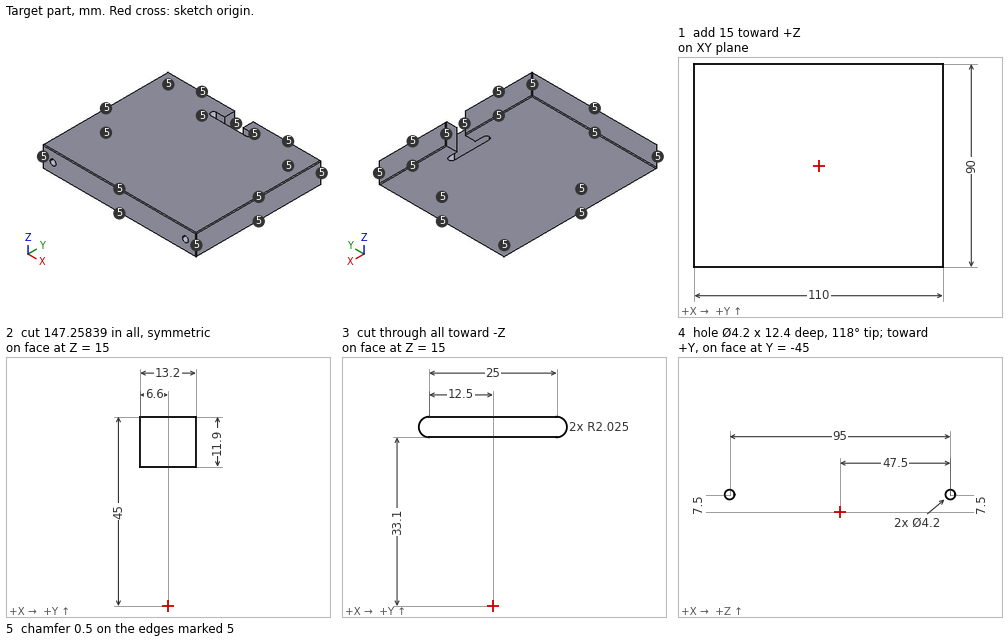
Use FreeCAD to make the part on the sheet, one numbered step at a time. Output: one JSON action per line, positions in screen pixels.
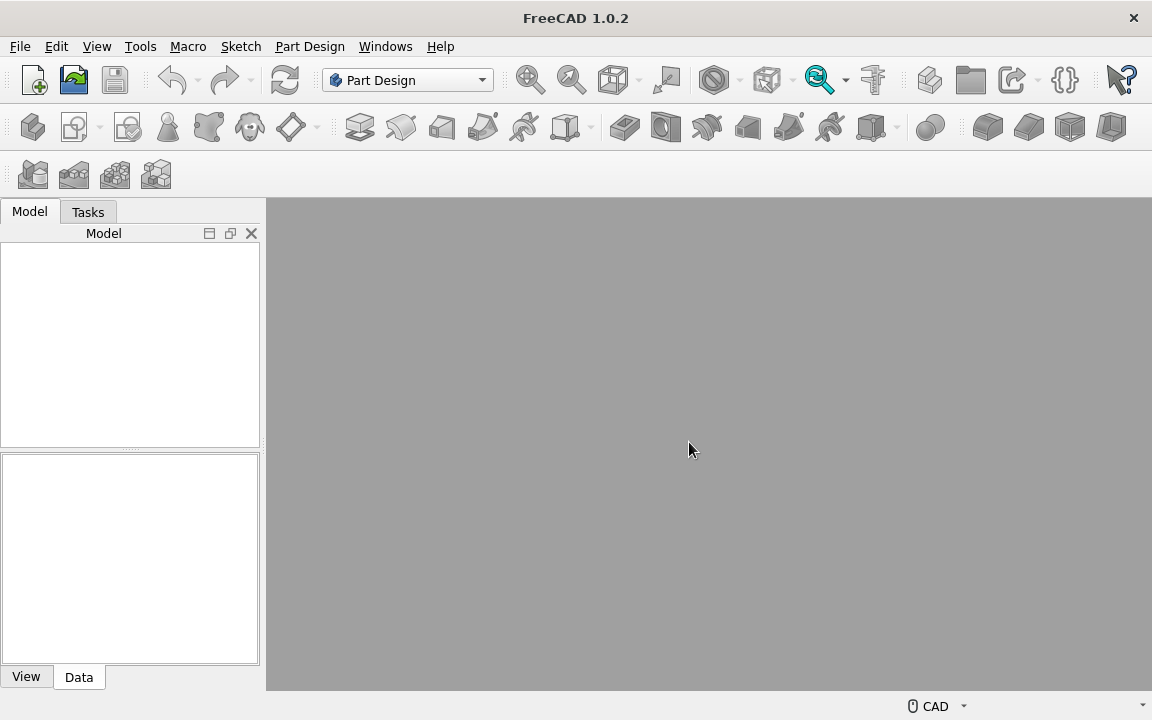
{"action": "left_click", "coordinate": [33, 80]}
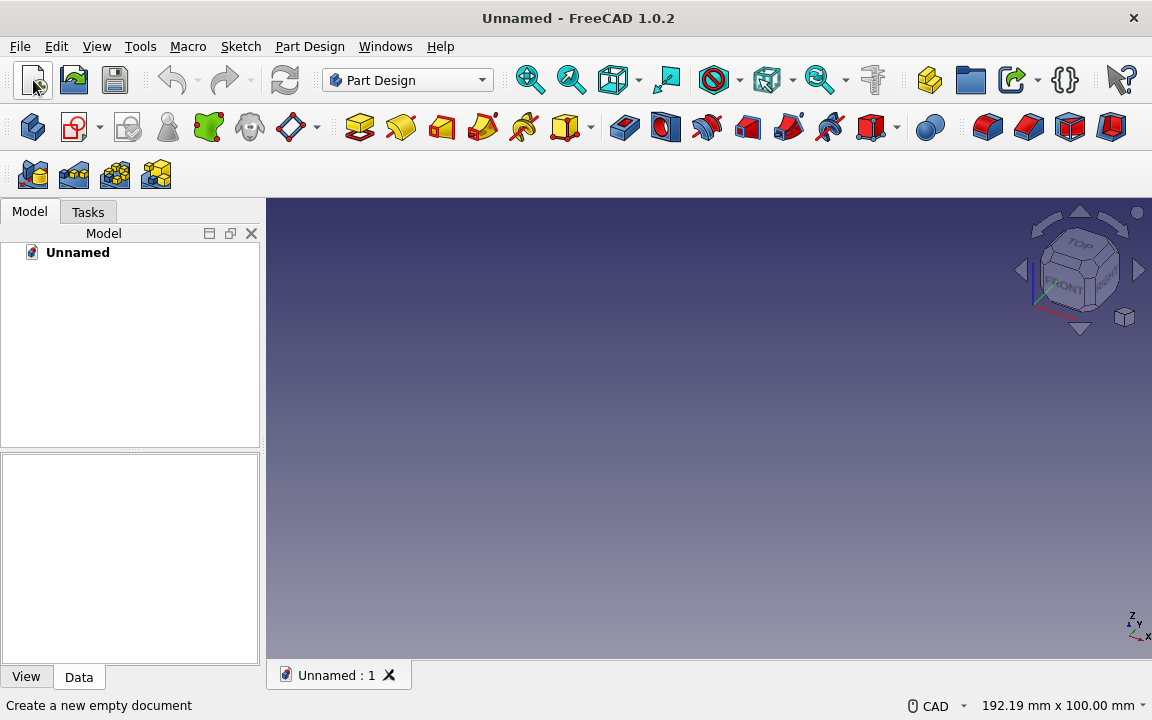
{"action": "left_click", "coordinate": [74, 128]}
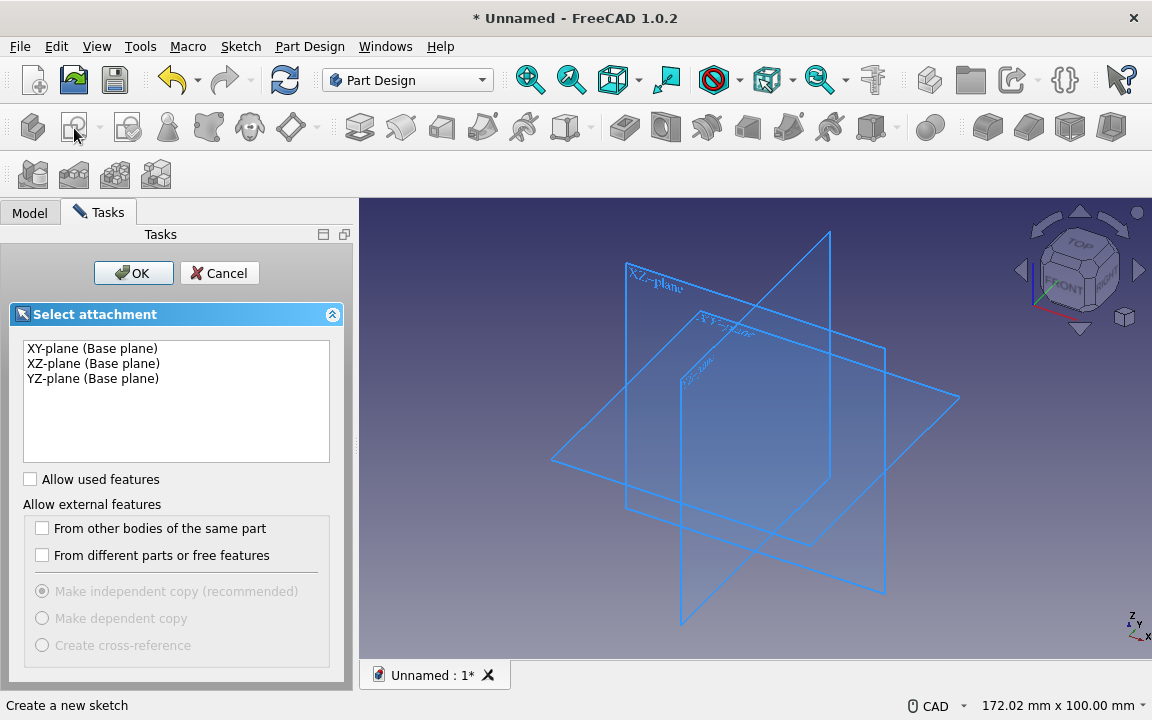
{"action": "left_click", "coordinate": [84, 348]}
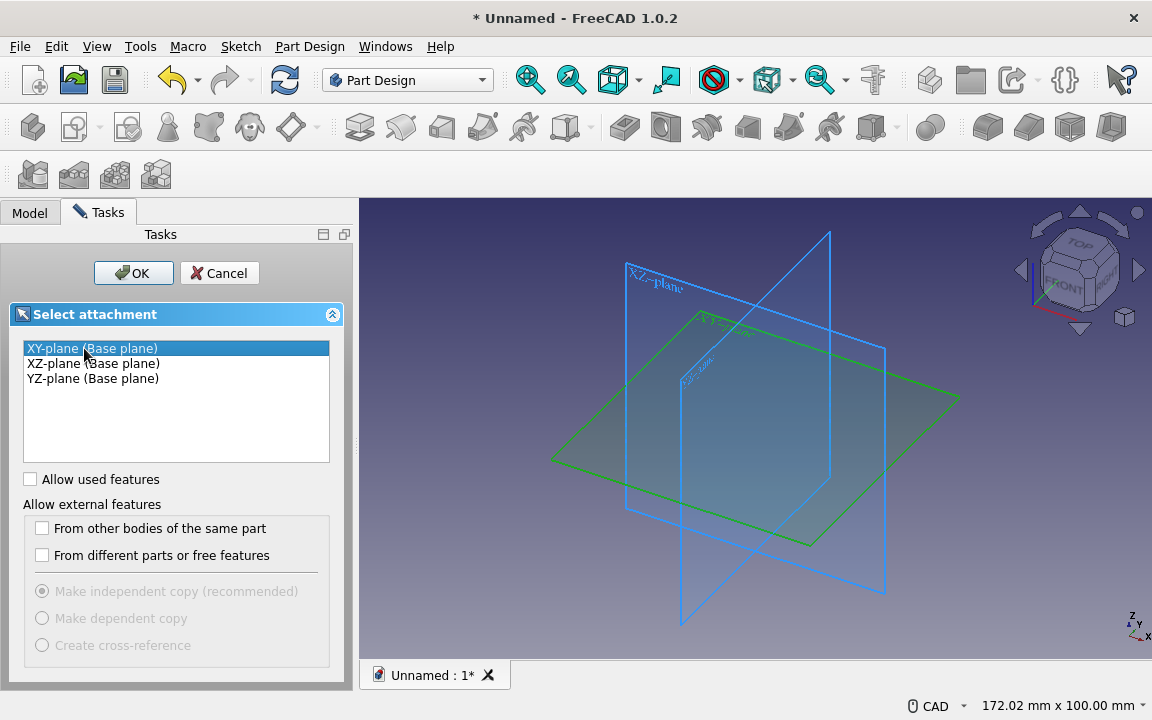
{"action": "left_click", "coordinate": [134, 273]}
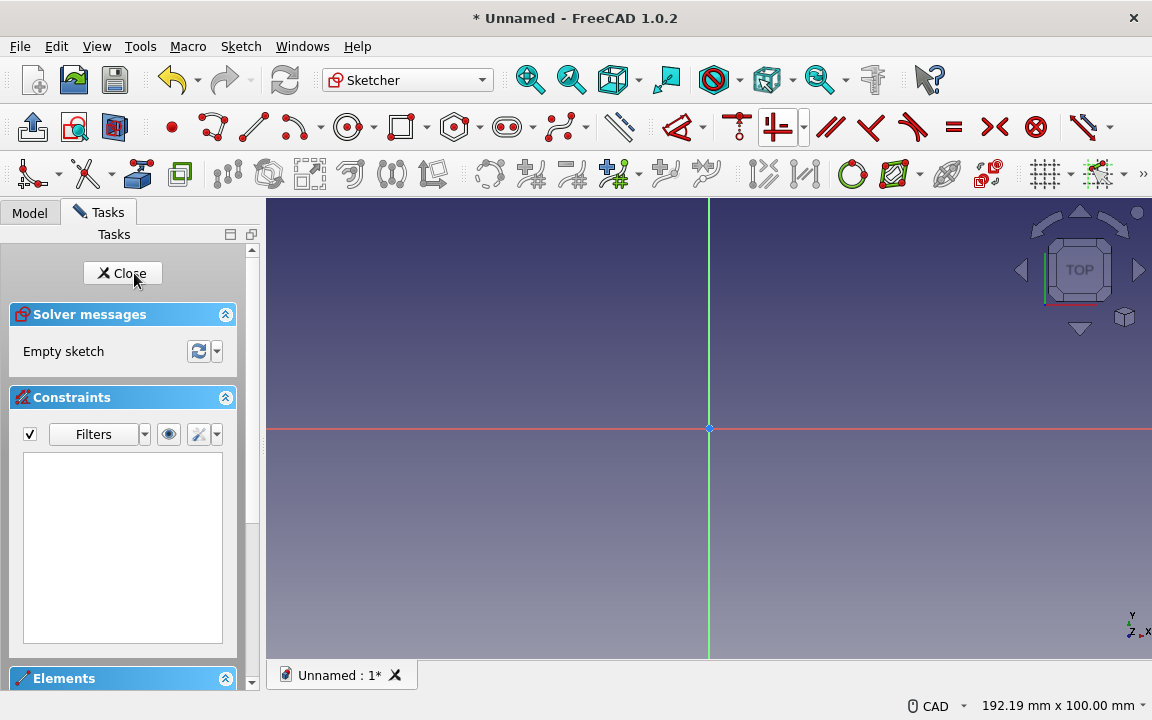
{"action": "scroll", "coordinate": [501, 429], "scroll_direction": "down", "scroll_amount": 2}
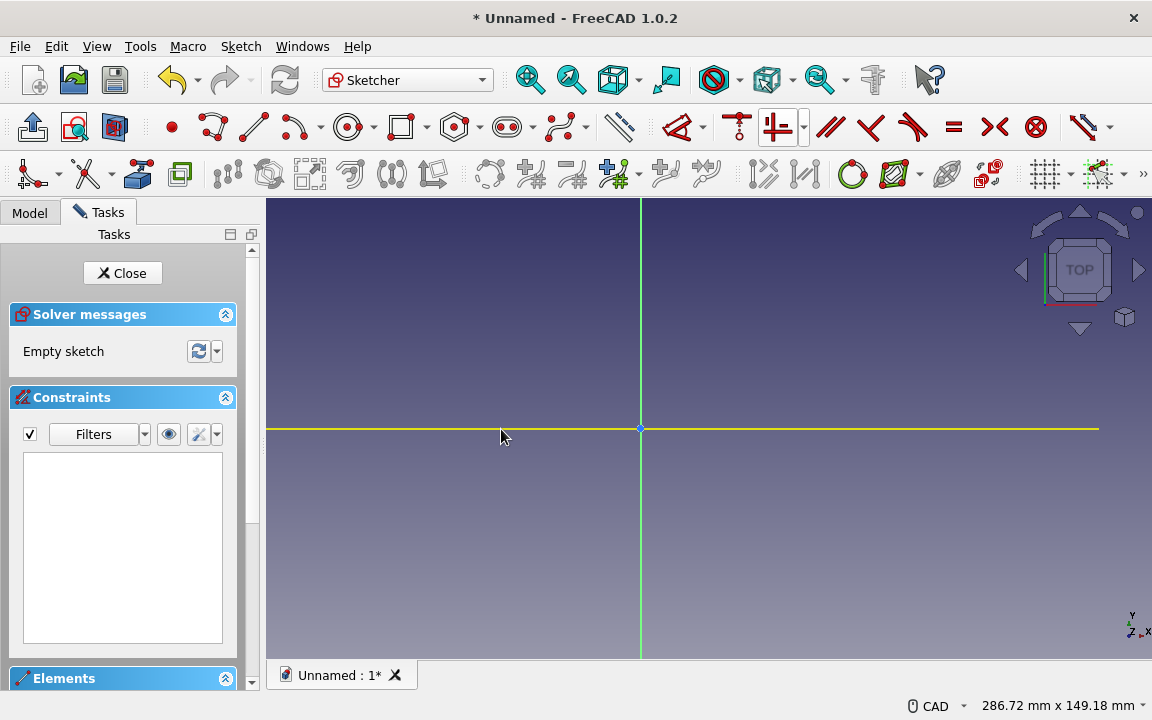
{"action": "key", "text": "g v"}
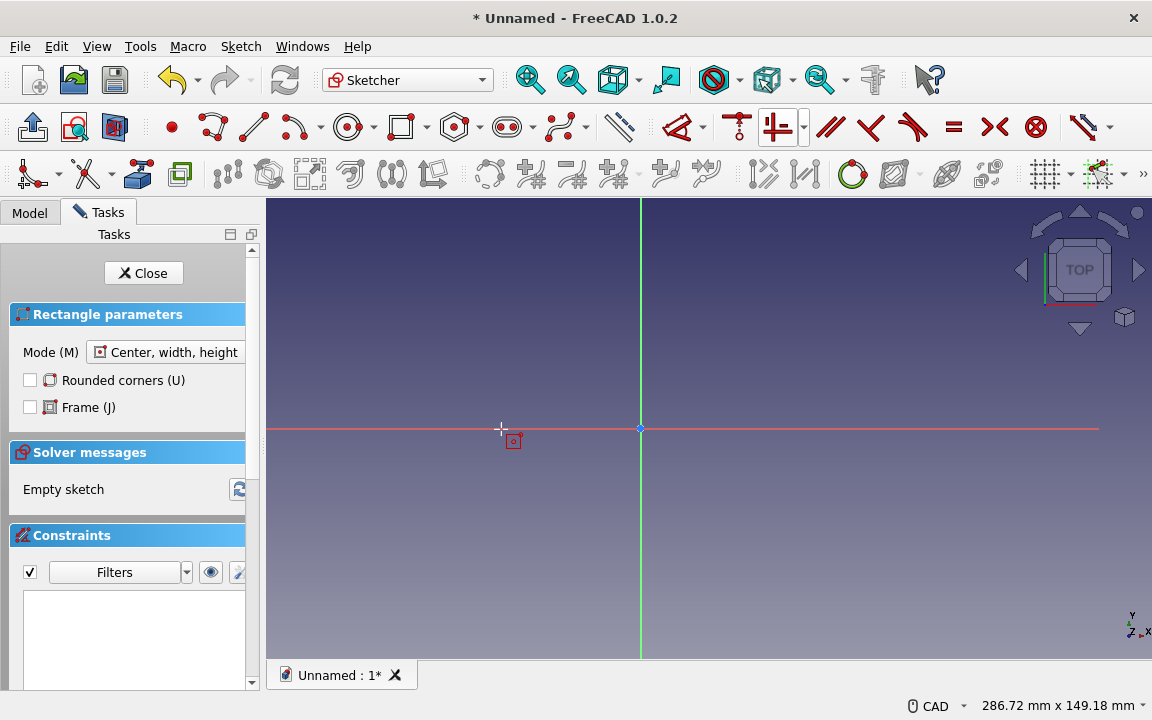
{"action": "left_click", "coordinate": [641, 429]}
{"action": "mouse_move", "coordinate": [810, 290]}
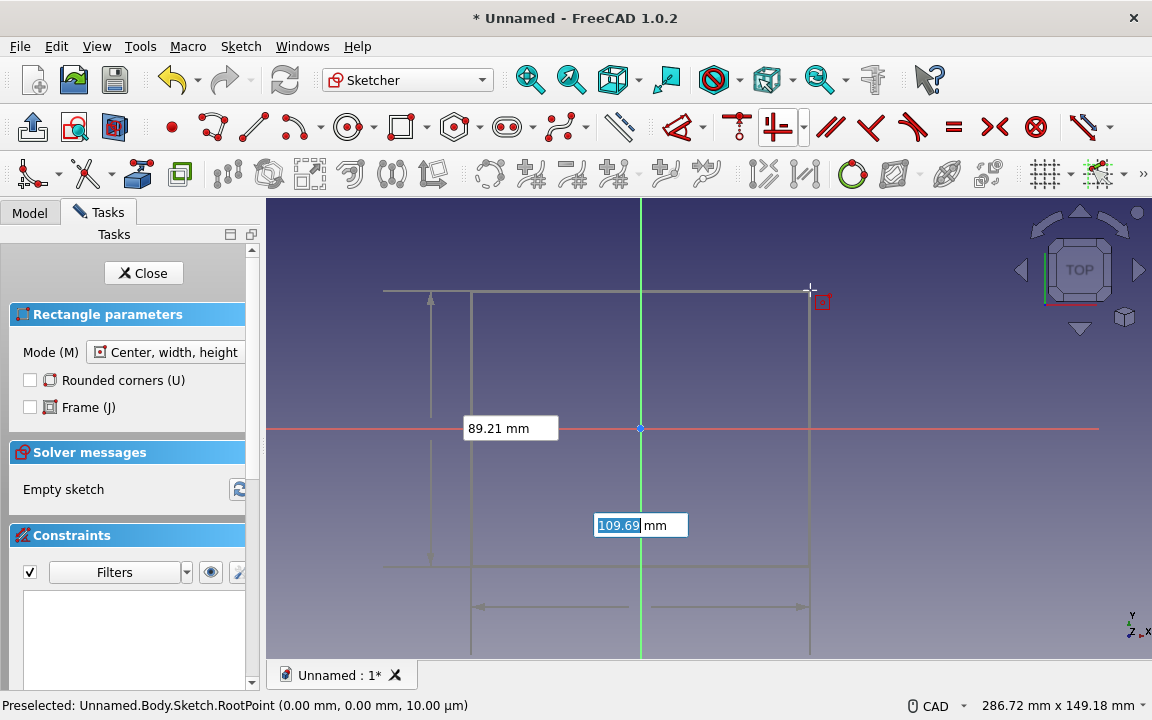
{"action": "type", "text": "110"}
{"action": "key", "text": "Tab"}
{"action": "type", "text": "90"}
{"action": "key", "text": "Return"}
{"action": "key", "text": "Escape"}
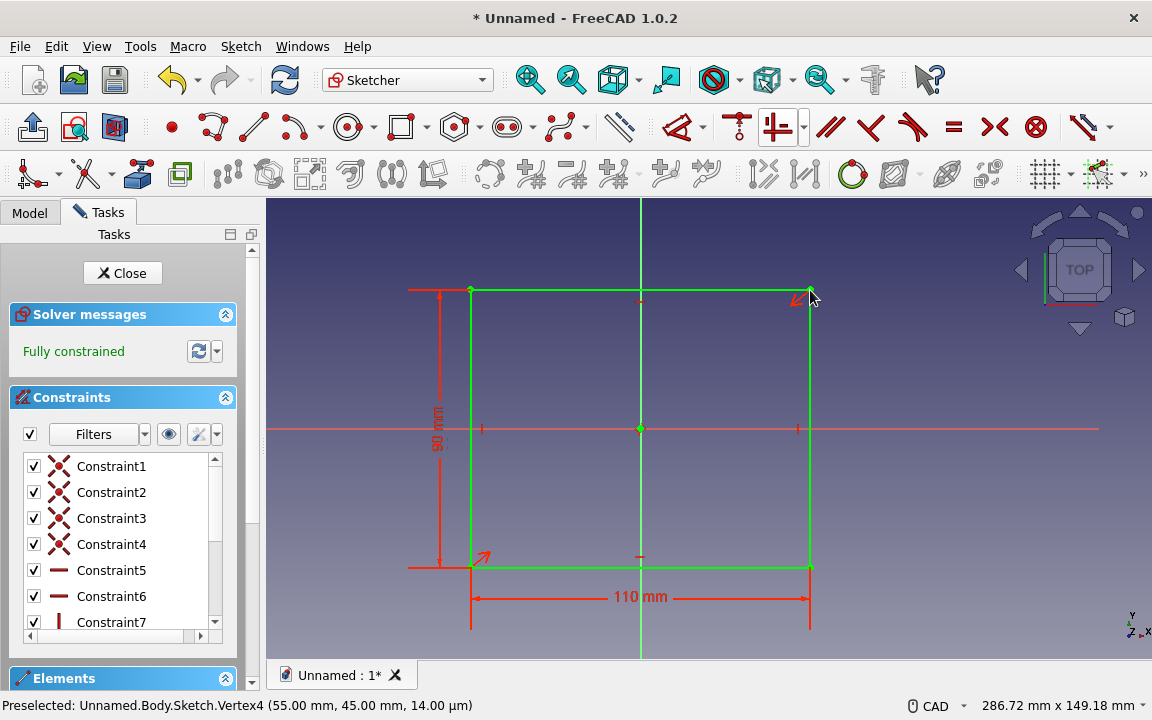
{"action": "left_click", "coordinate": [123, 273]}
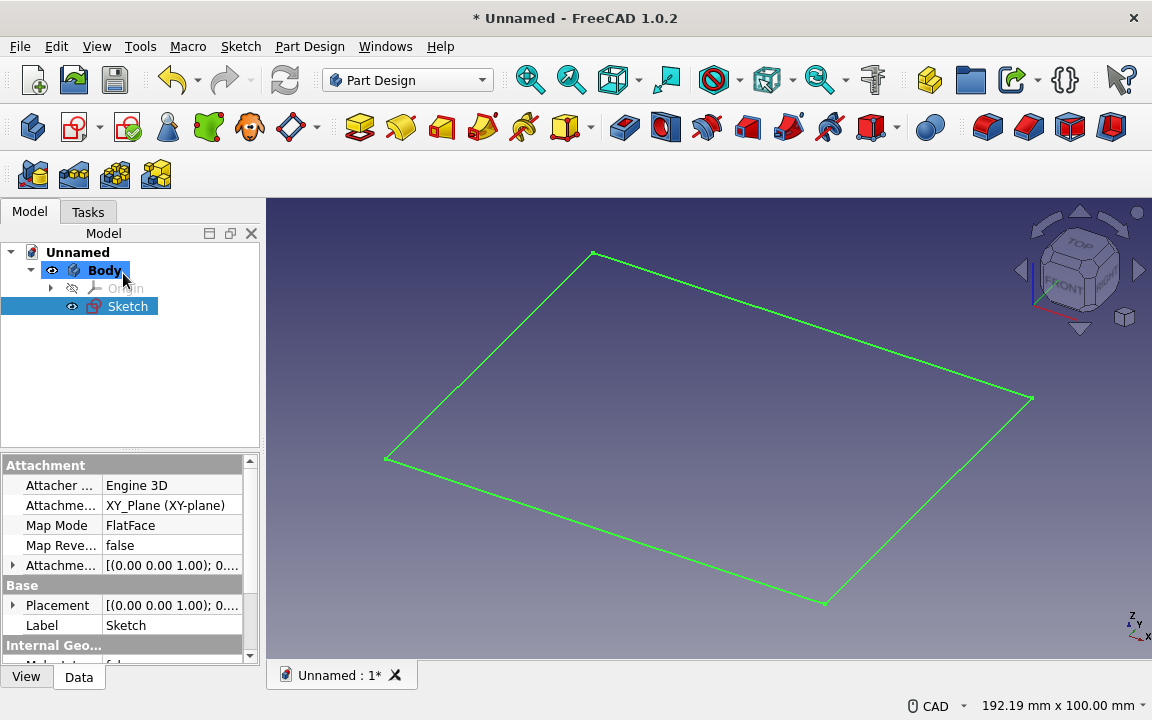
{"action": "left_click", "coordinate": [360, 128]}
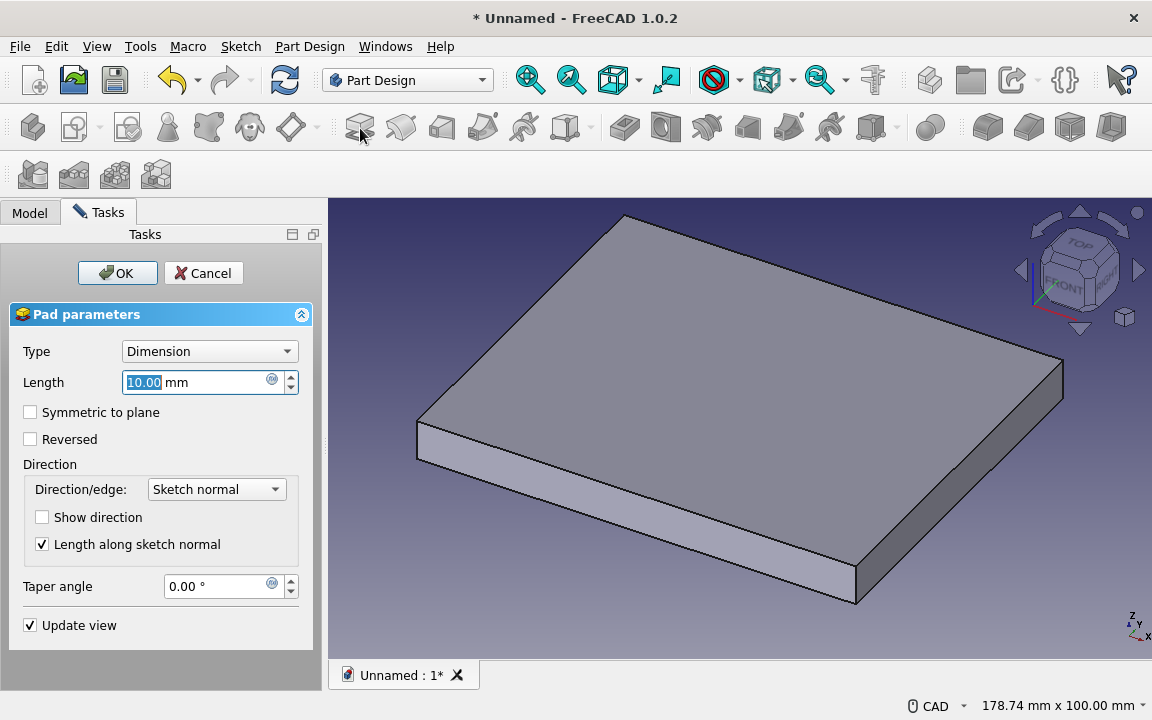
{"action": "type", "text": "15"}
{"action": "key", "text": "Tab"}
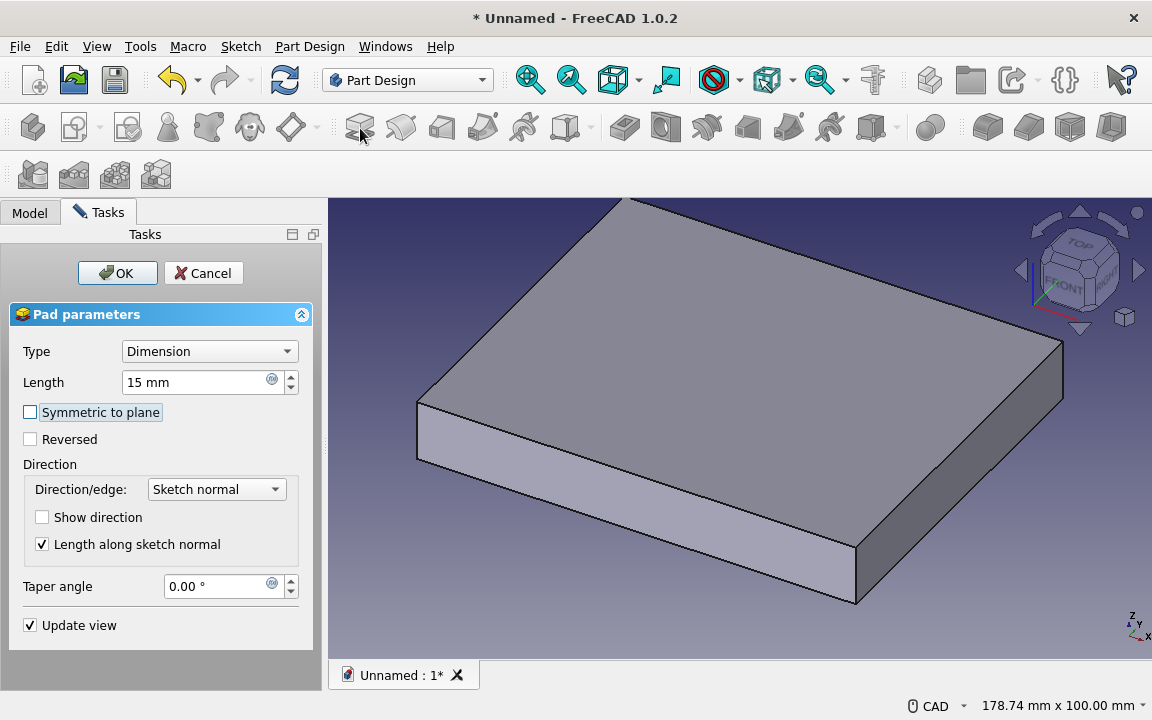
{"action": "left_click", "coordinate": [118, 273]}